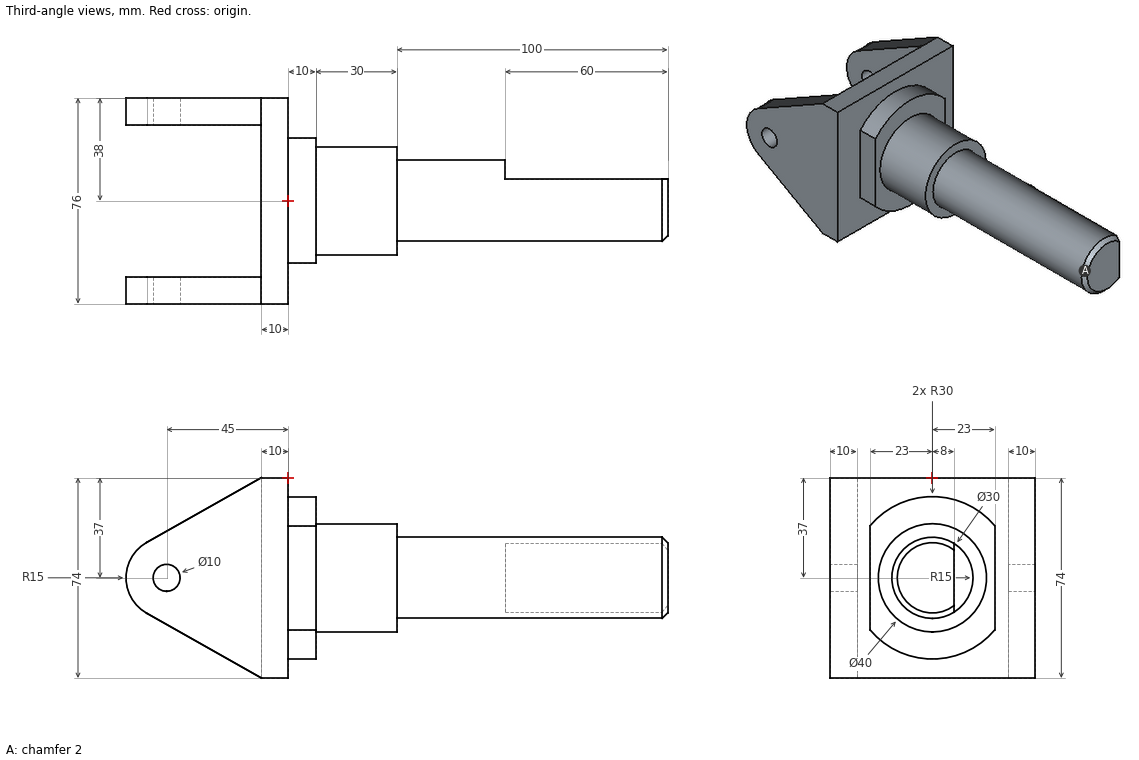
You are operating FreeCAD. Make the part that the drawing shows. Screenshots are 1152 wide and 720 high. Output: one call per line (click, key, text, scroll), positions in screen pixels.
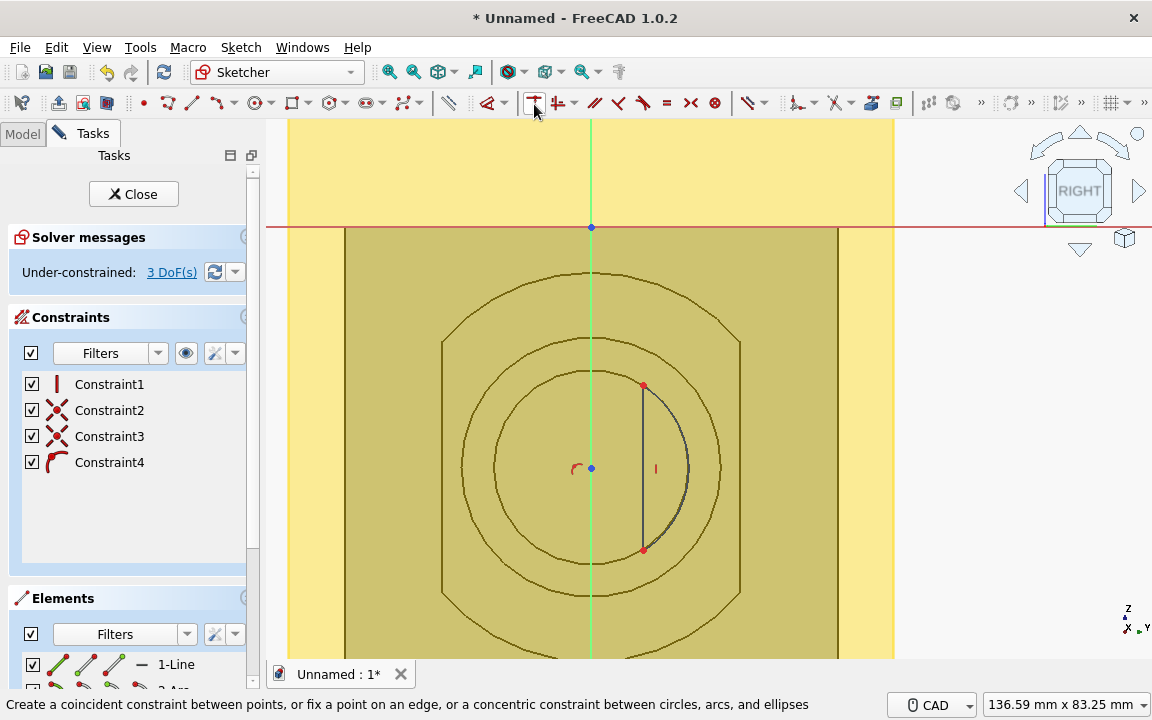
click(488, 104)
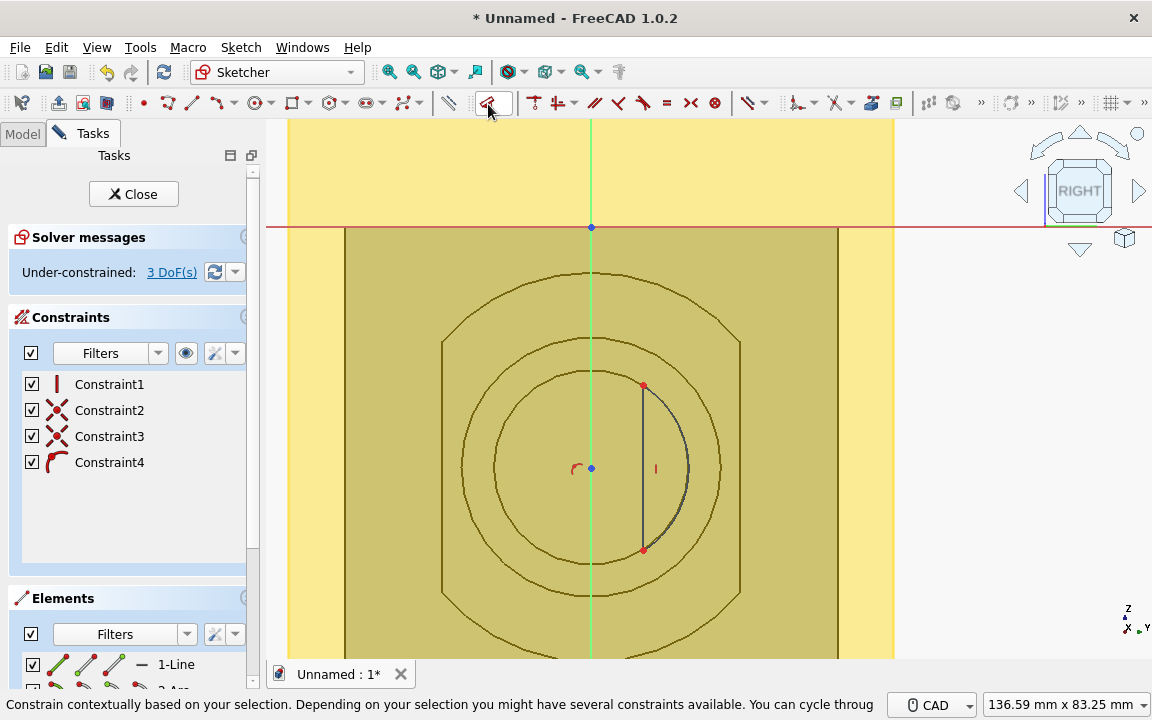
click(681, 507)
click(710, 520)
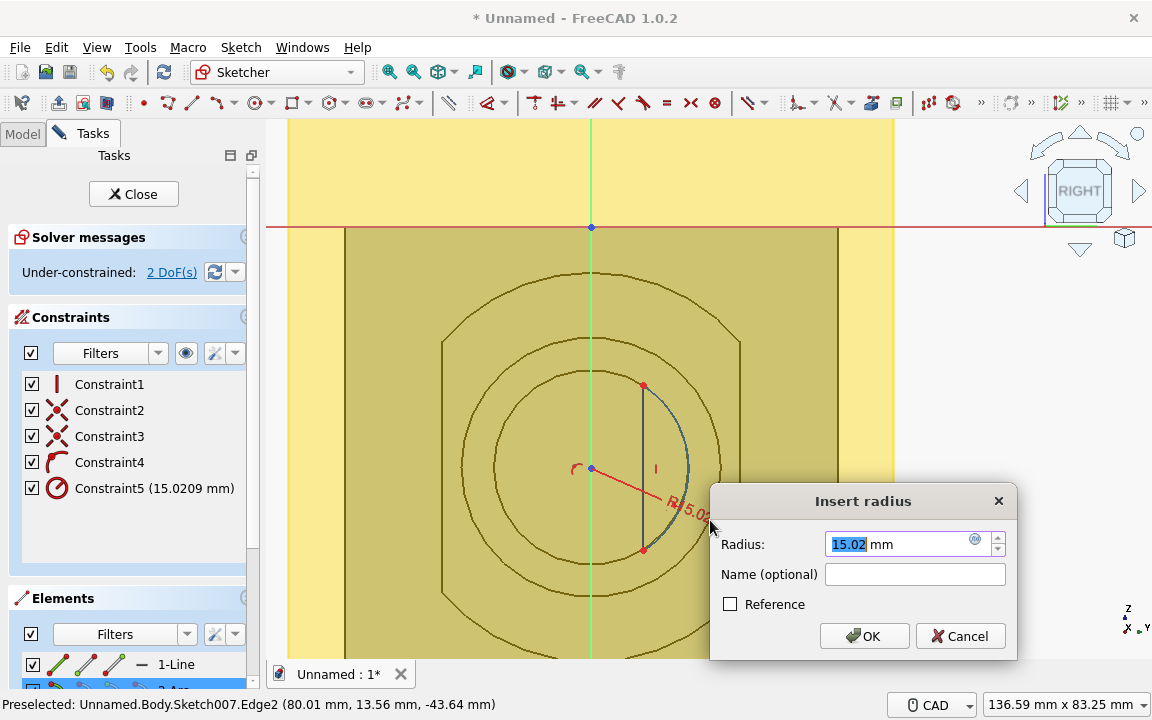
text(15)
key(Return)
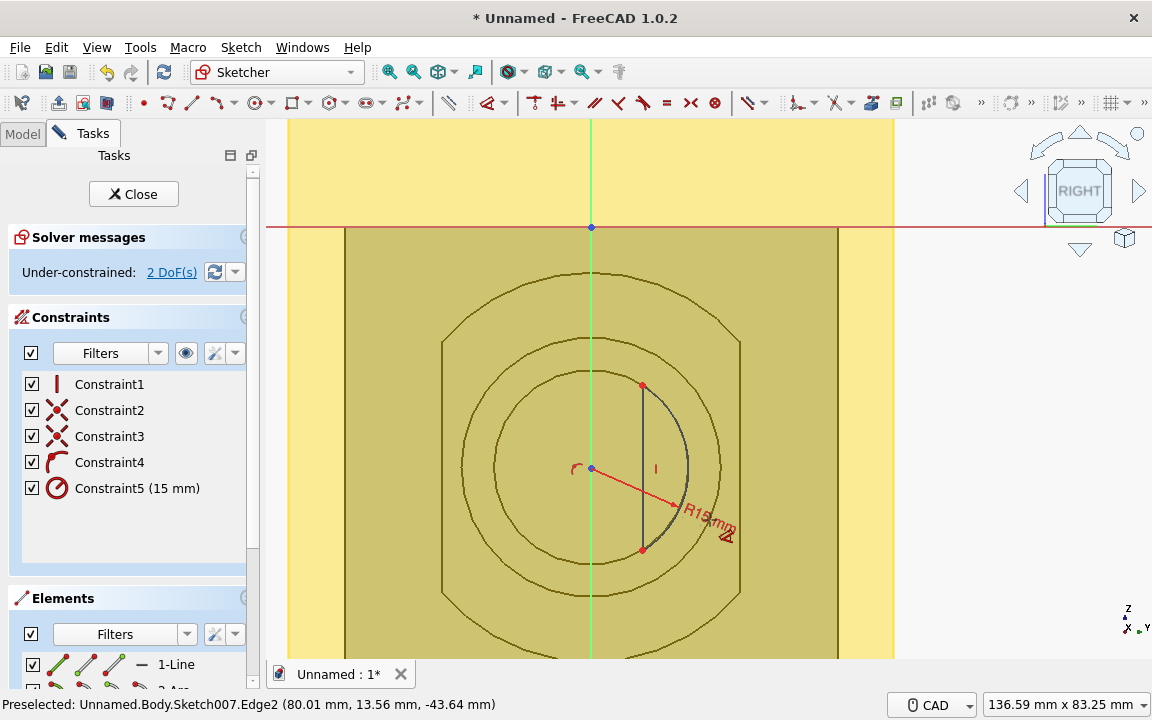
click(643, 386)
click(617, 193)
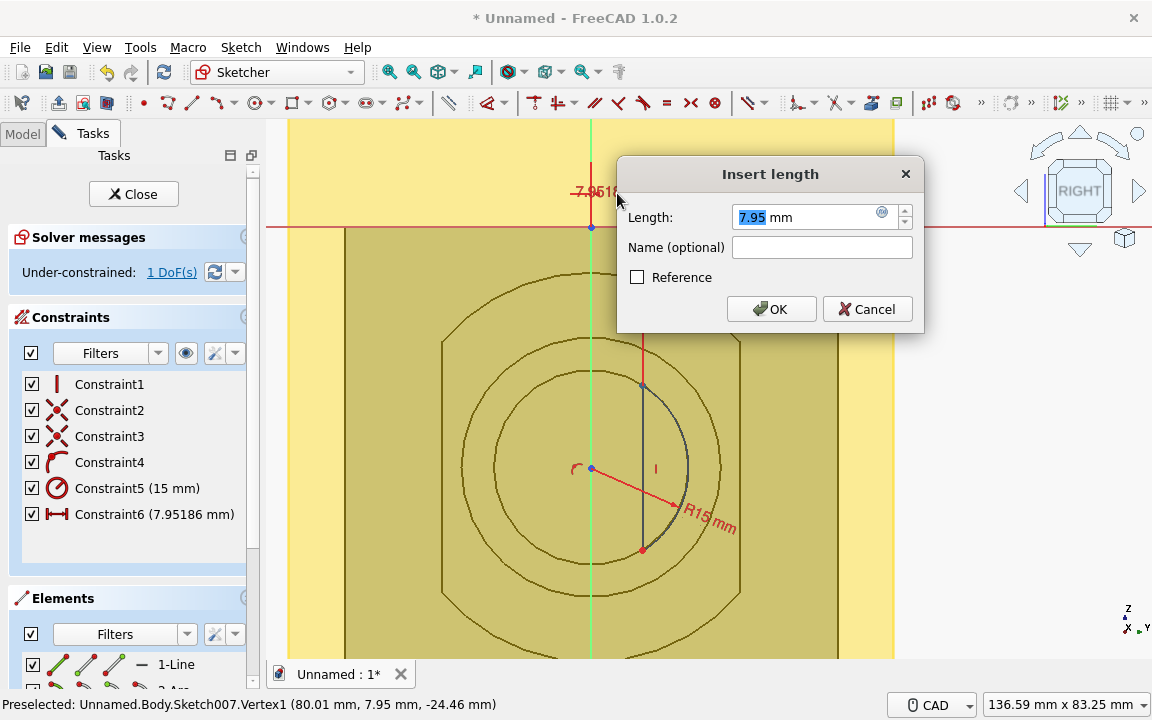
text(8)
key(Return)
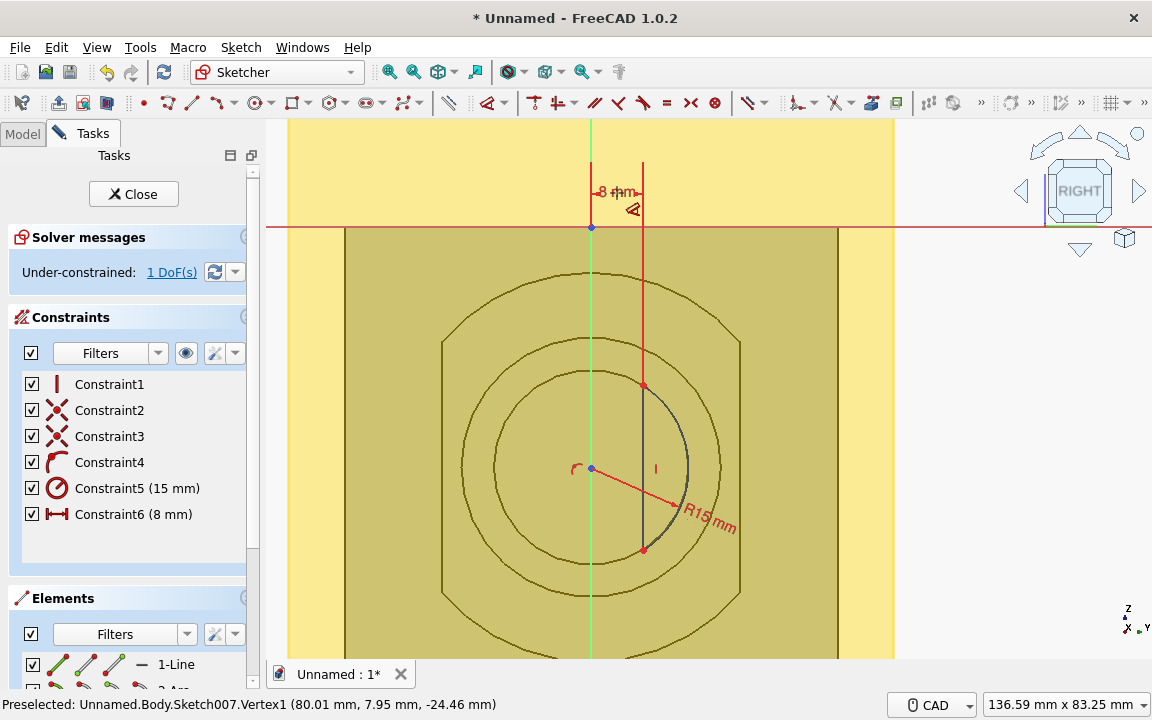
click(591, 468)
click(557, 348)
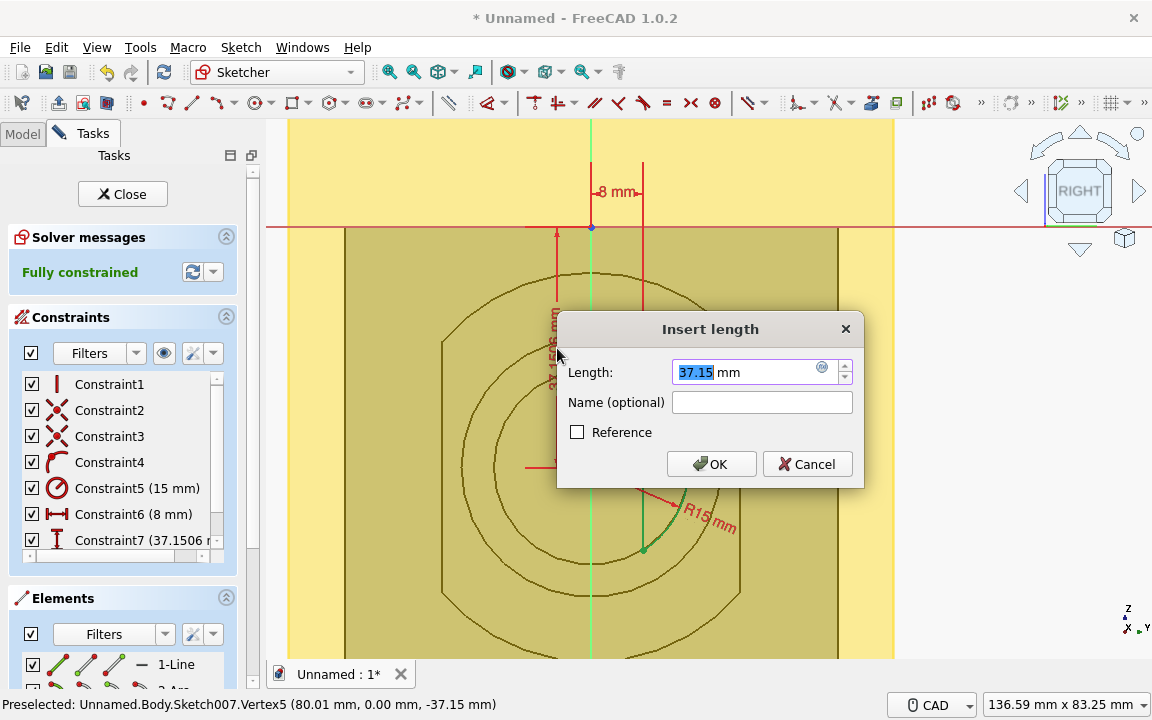
text(37)
key(Return)
key(Escape)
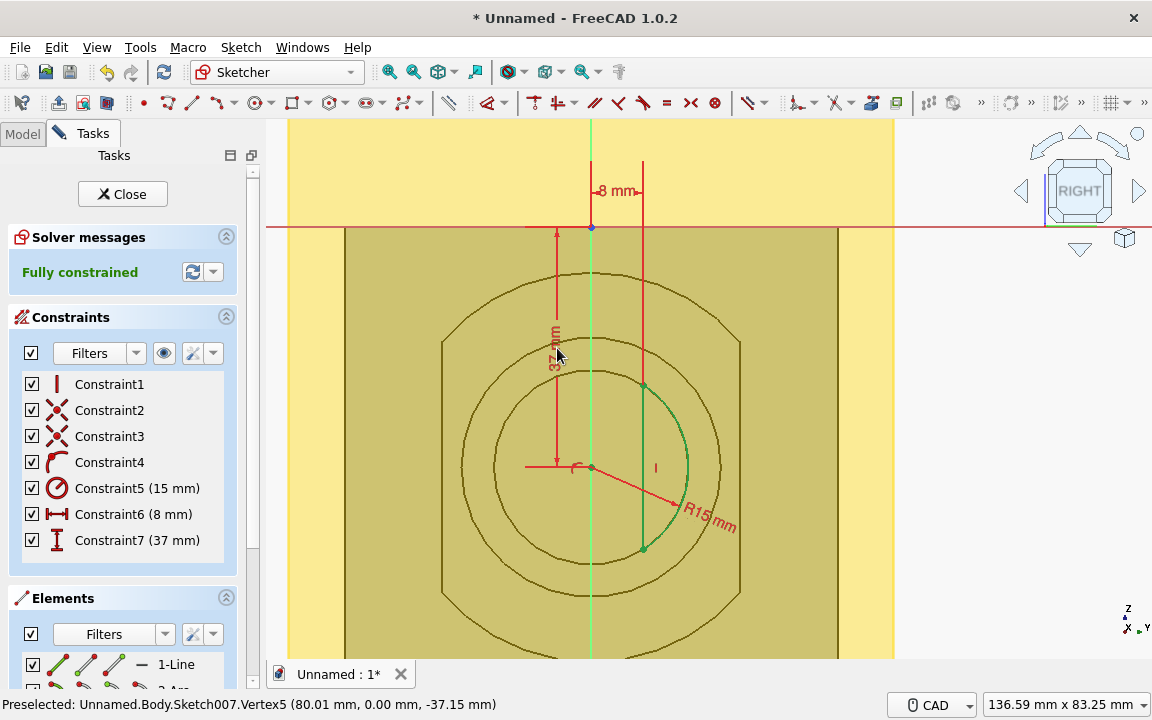
click(123, 194)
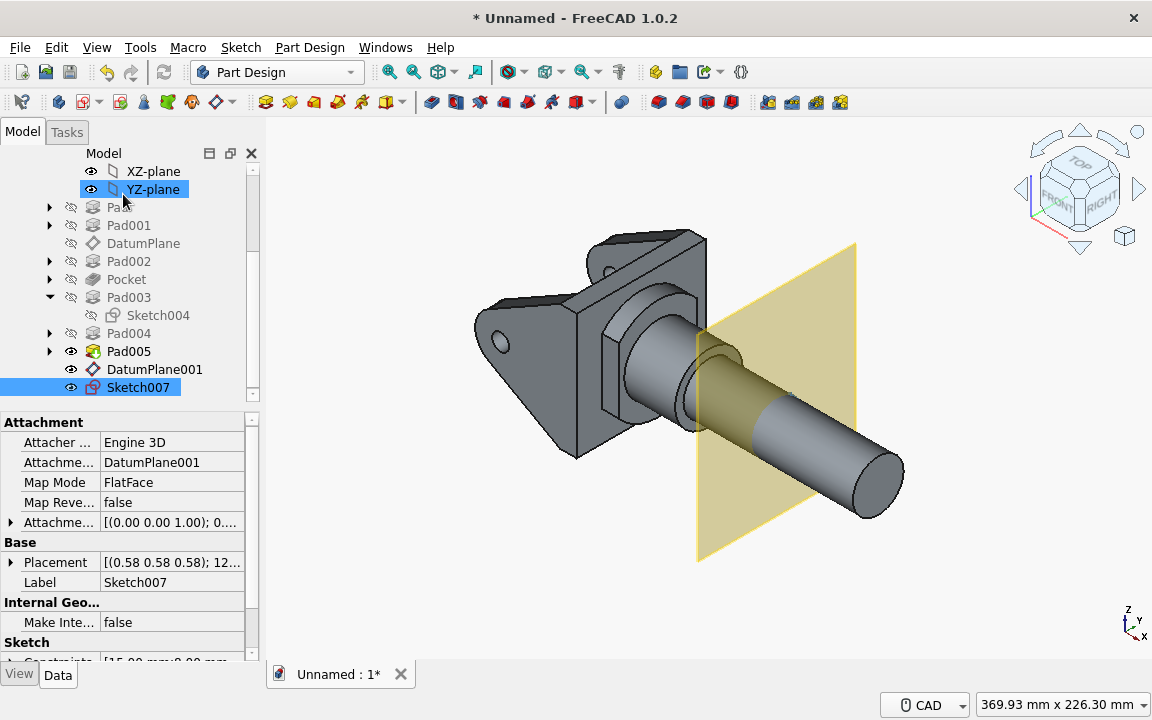
click(432, 102)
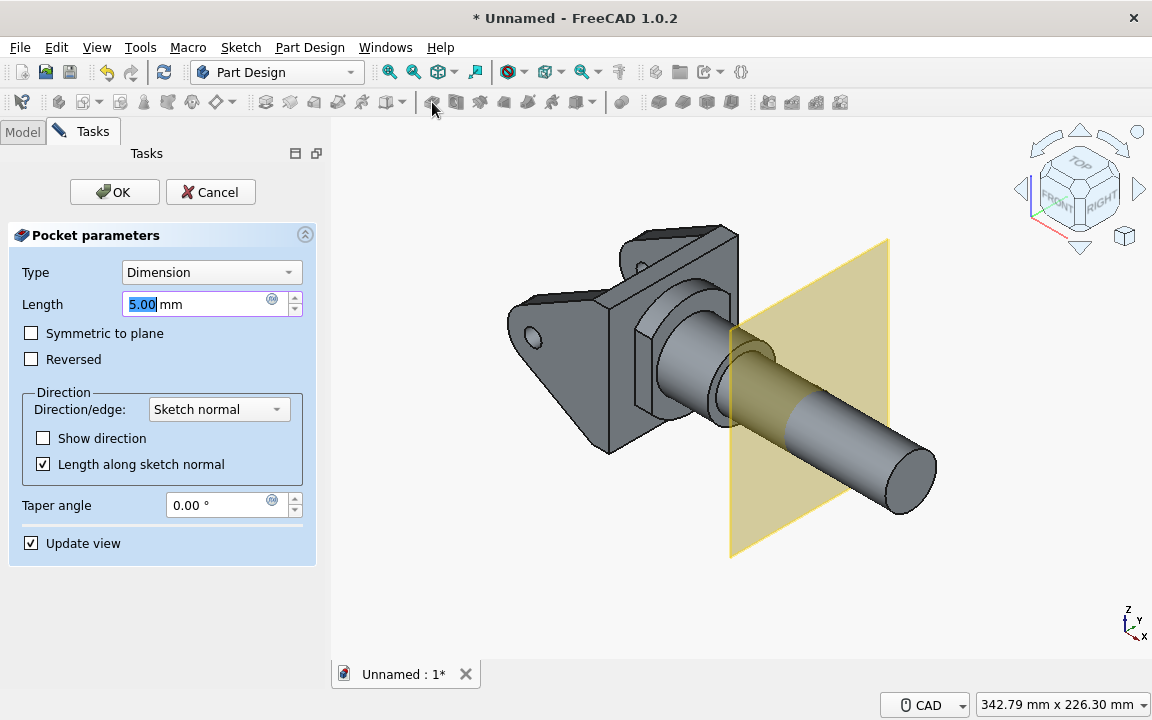
text(60)
key(Tab)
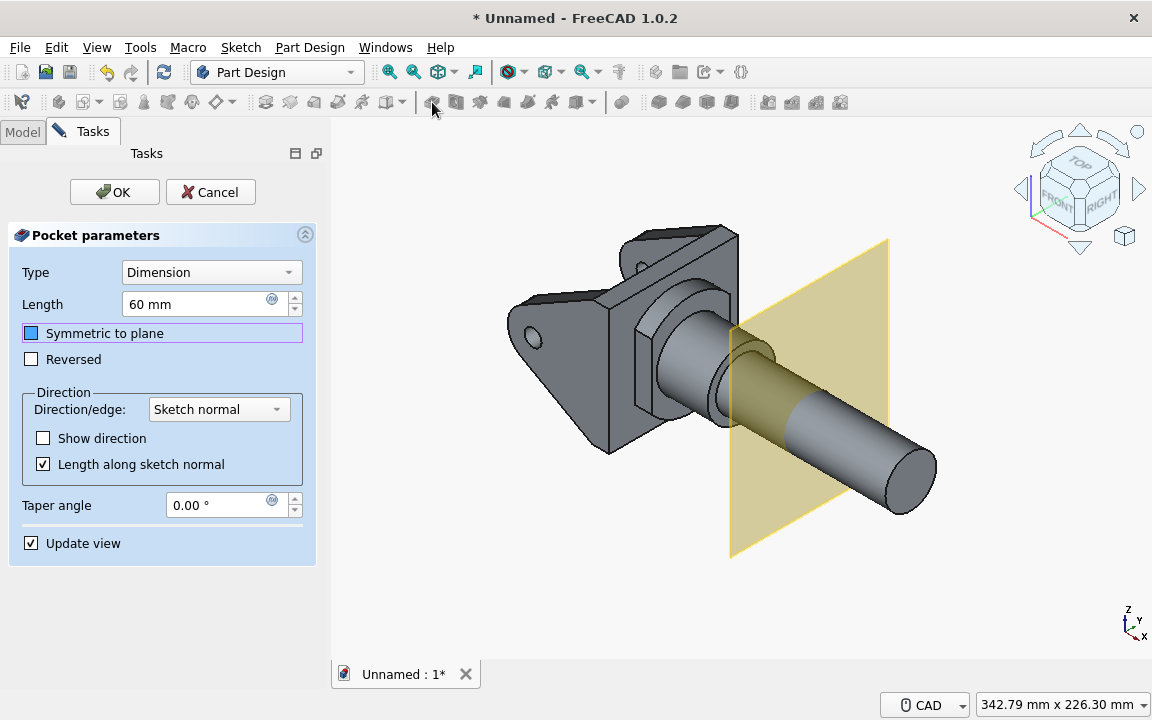
click(30, 359)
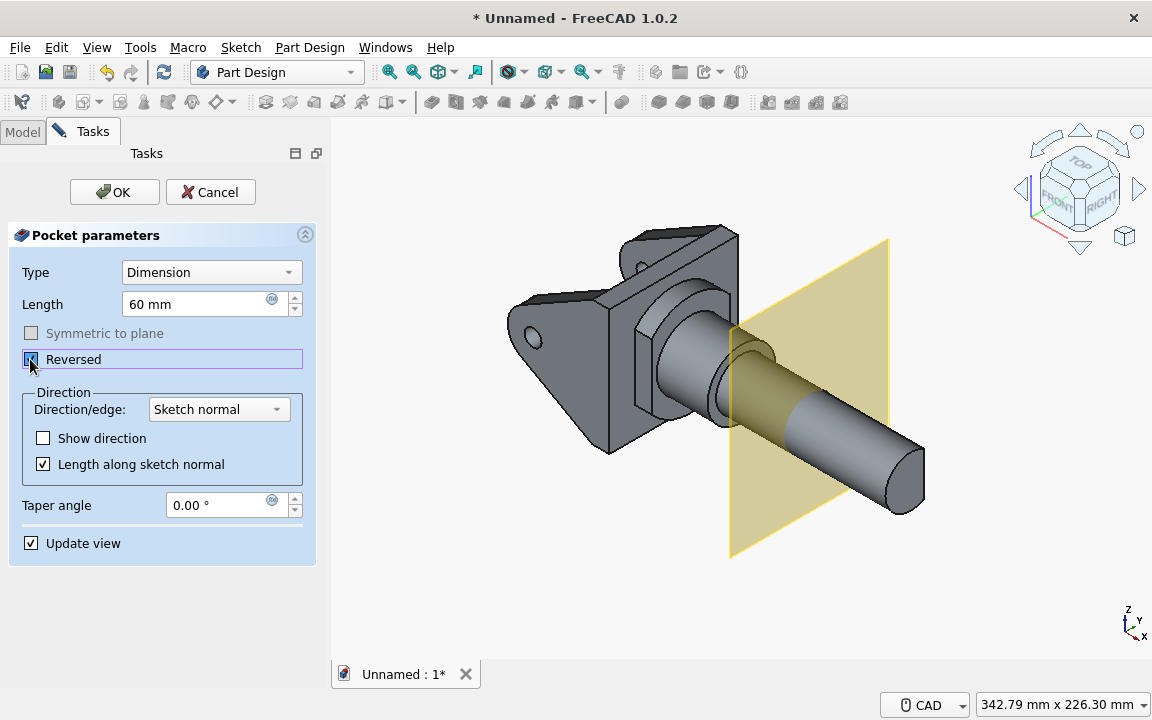
click(115, 192)